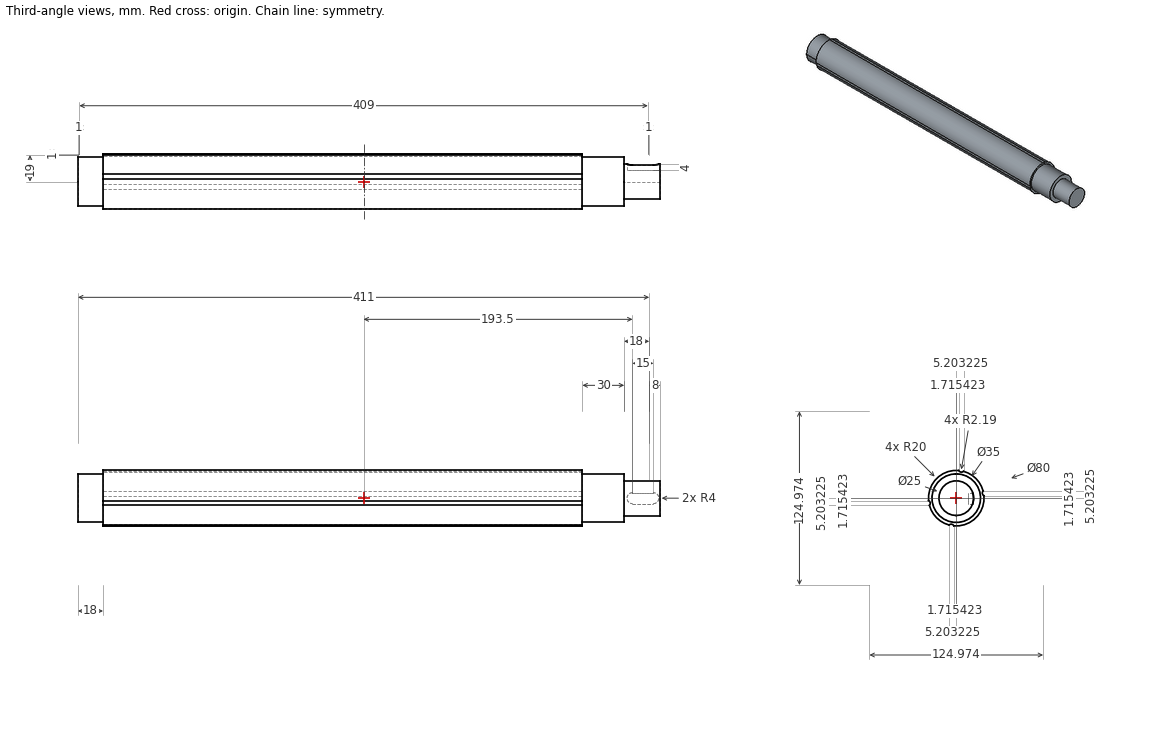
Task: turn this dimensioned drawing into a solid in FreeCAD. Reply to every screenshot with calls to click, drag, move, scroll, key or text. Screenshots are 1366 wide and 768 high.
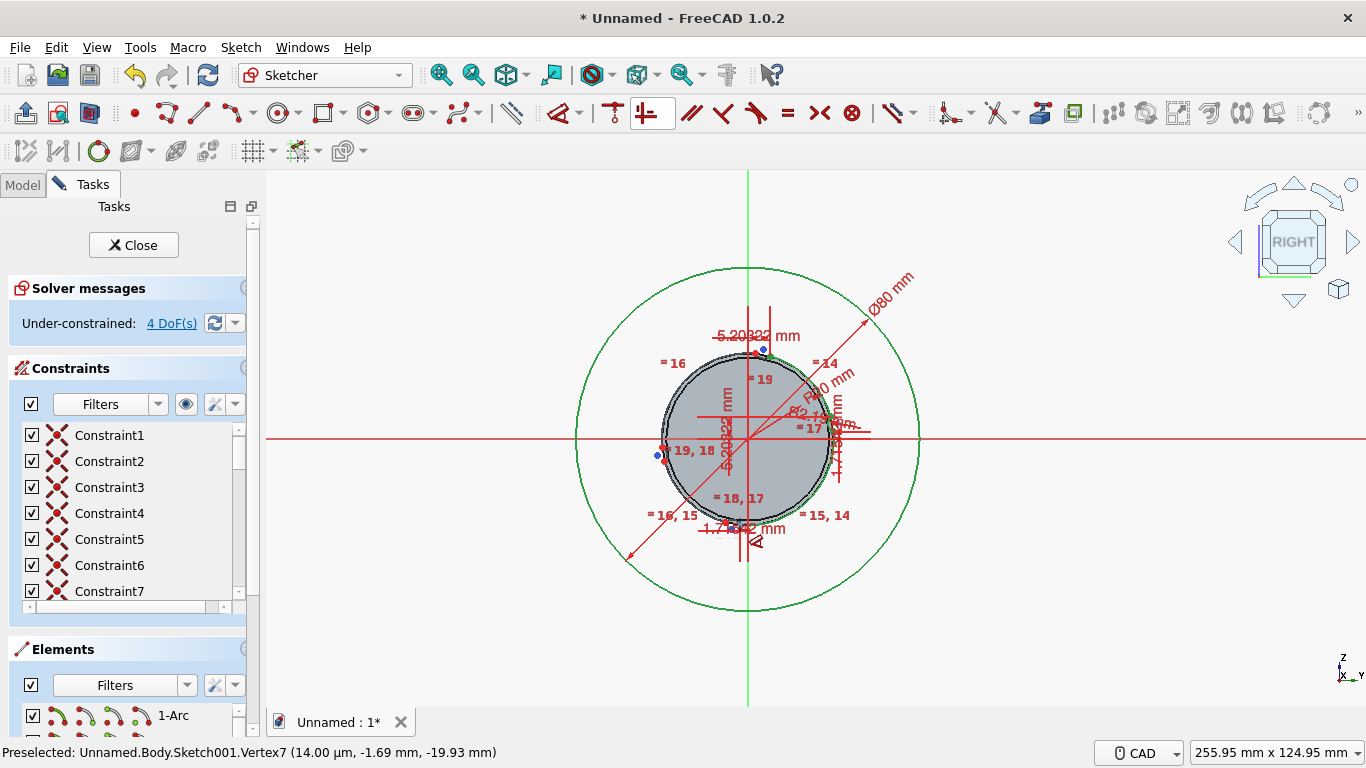
scroll(725, 522, up, 3)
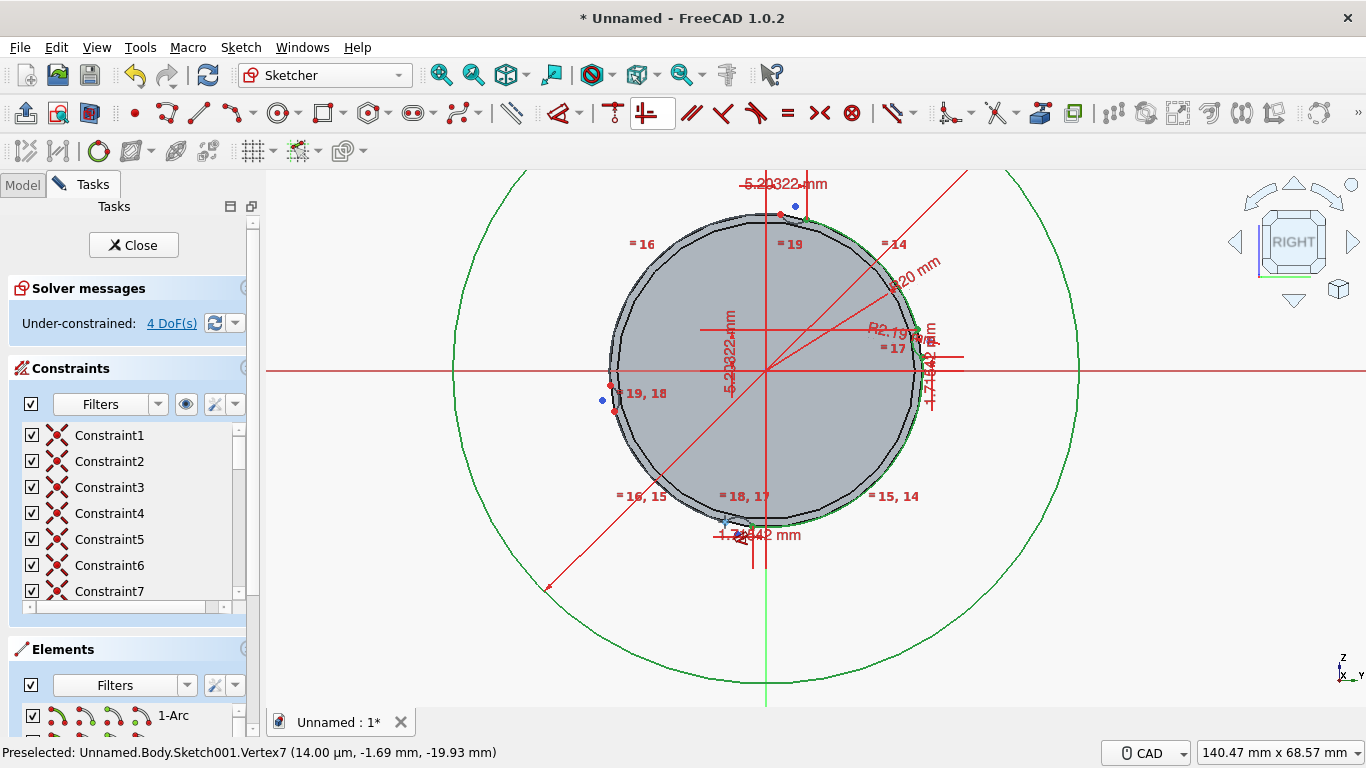
click(726, 522)
click(746, 580)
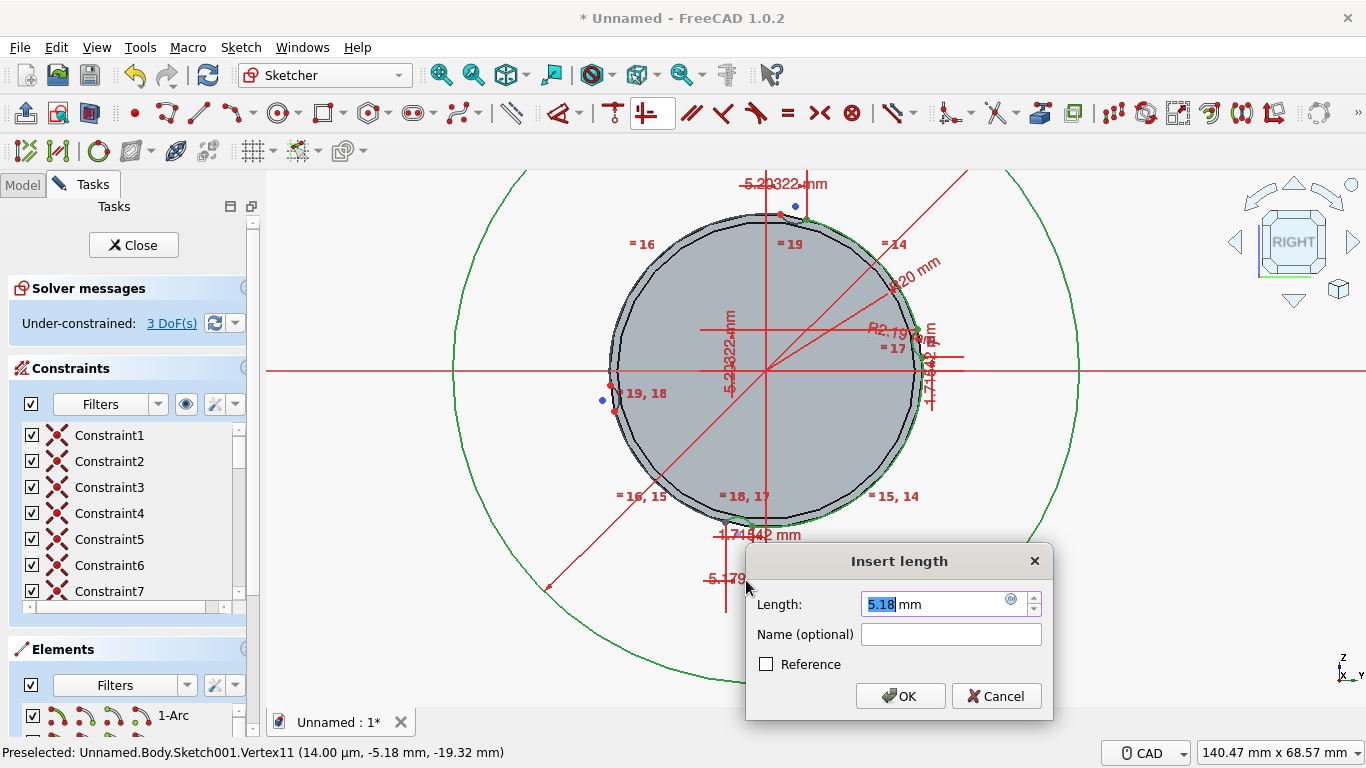
text(5.203225)
key(Return)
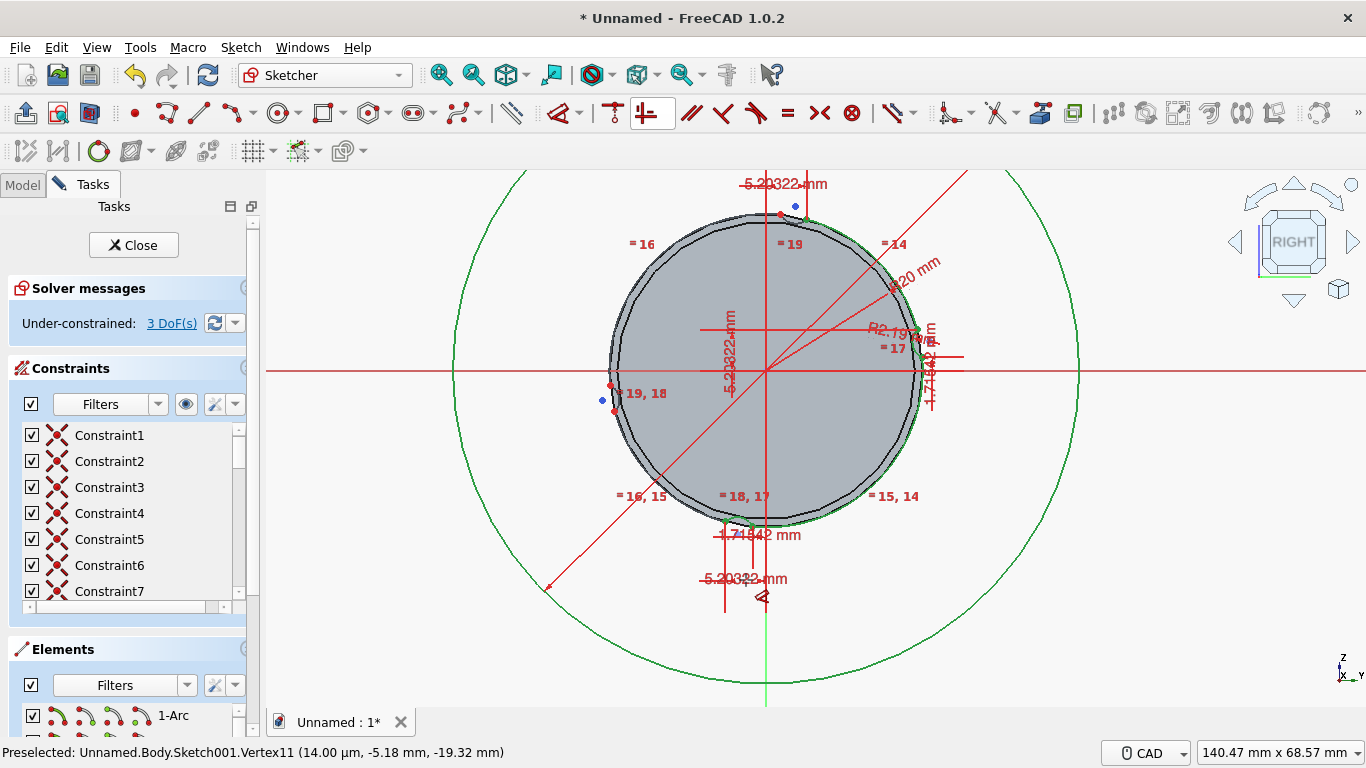
click(615, 412)
click(581, 391)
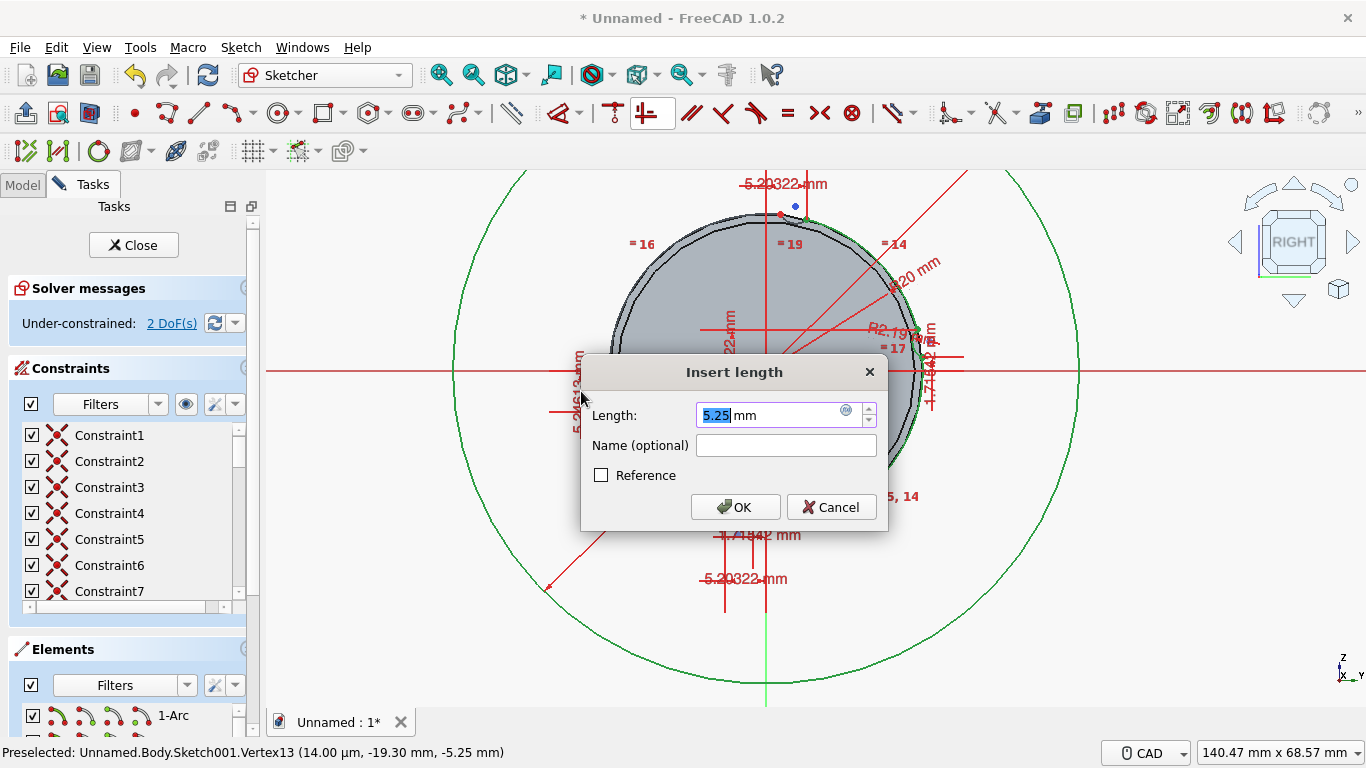
text(5.203225)
key(Return)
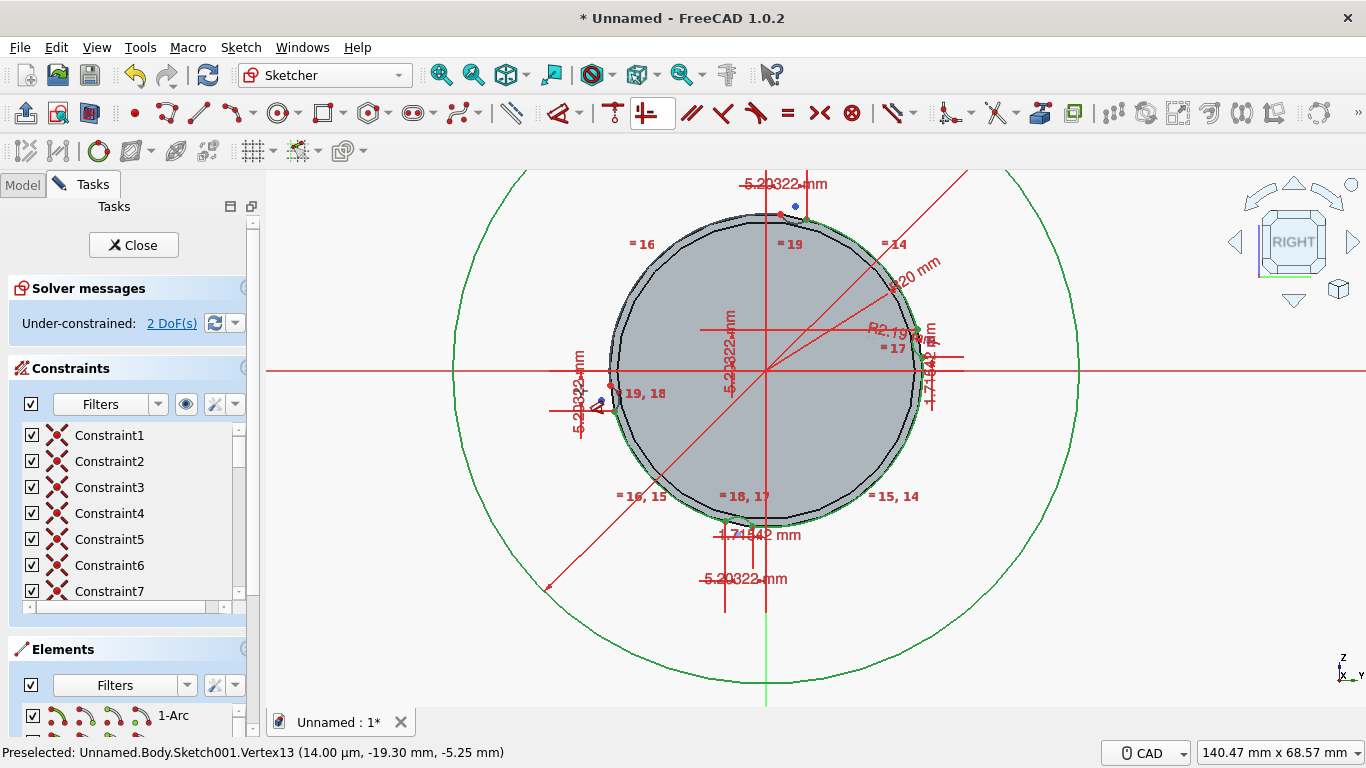
scroll(610, 385, up, 6)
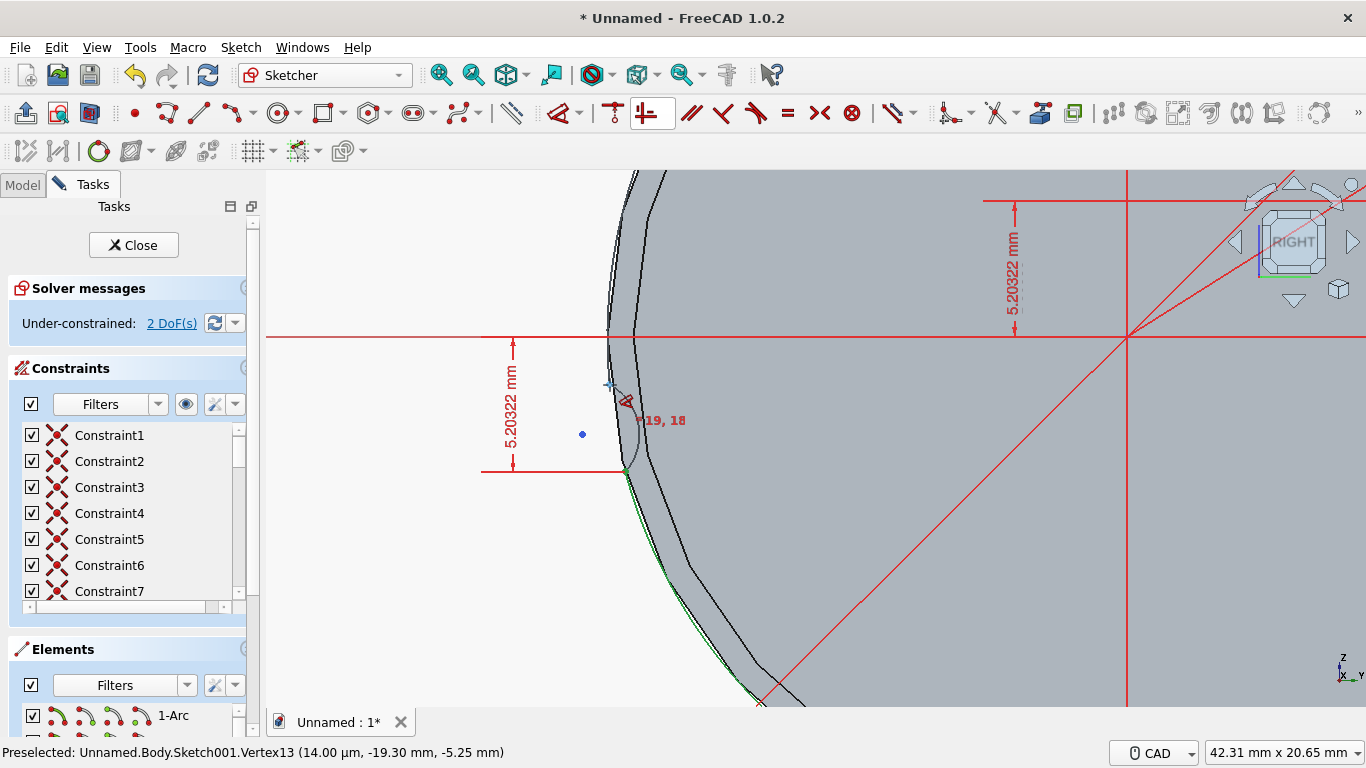
click(610, 385)
click(576, 361)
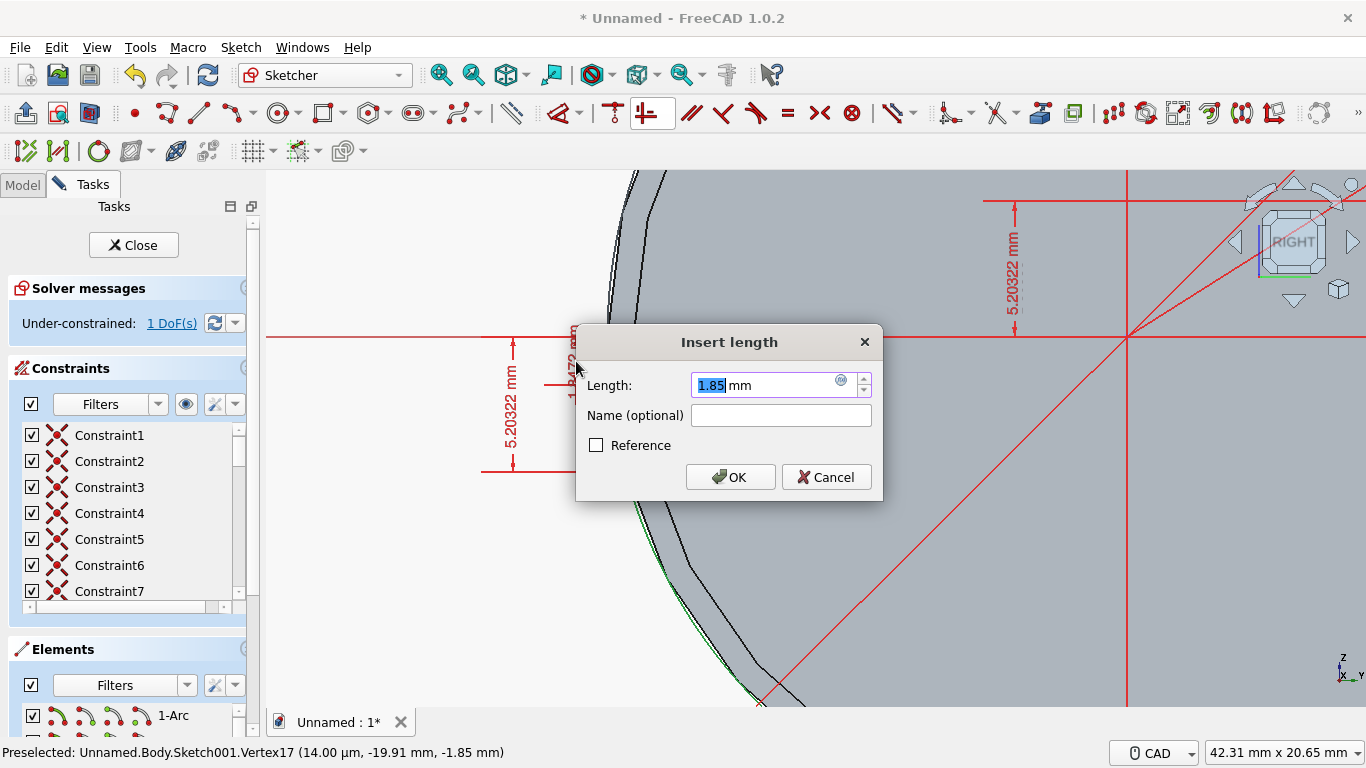
text(1.715423)
key(Return)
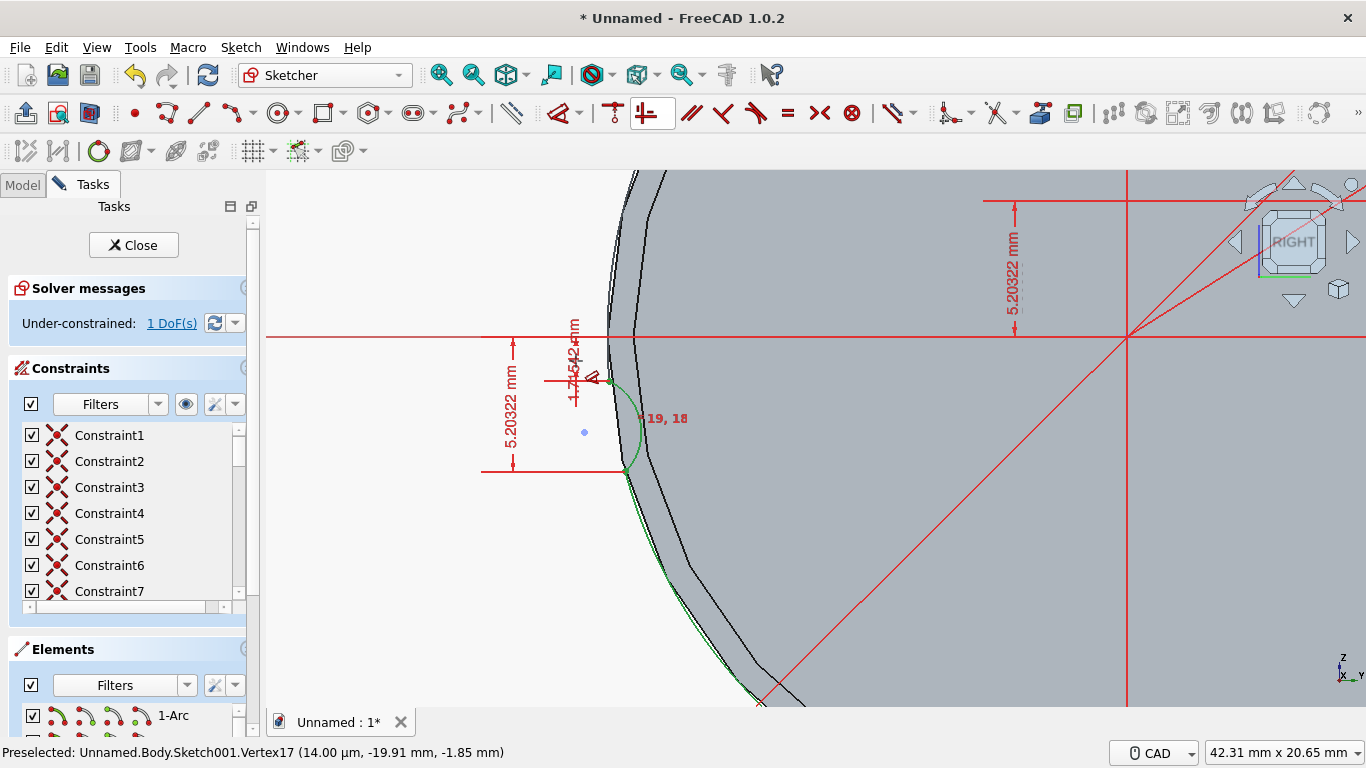
scroll(672, 459, down, 9)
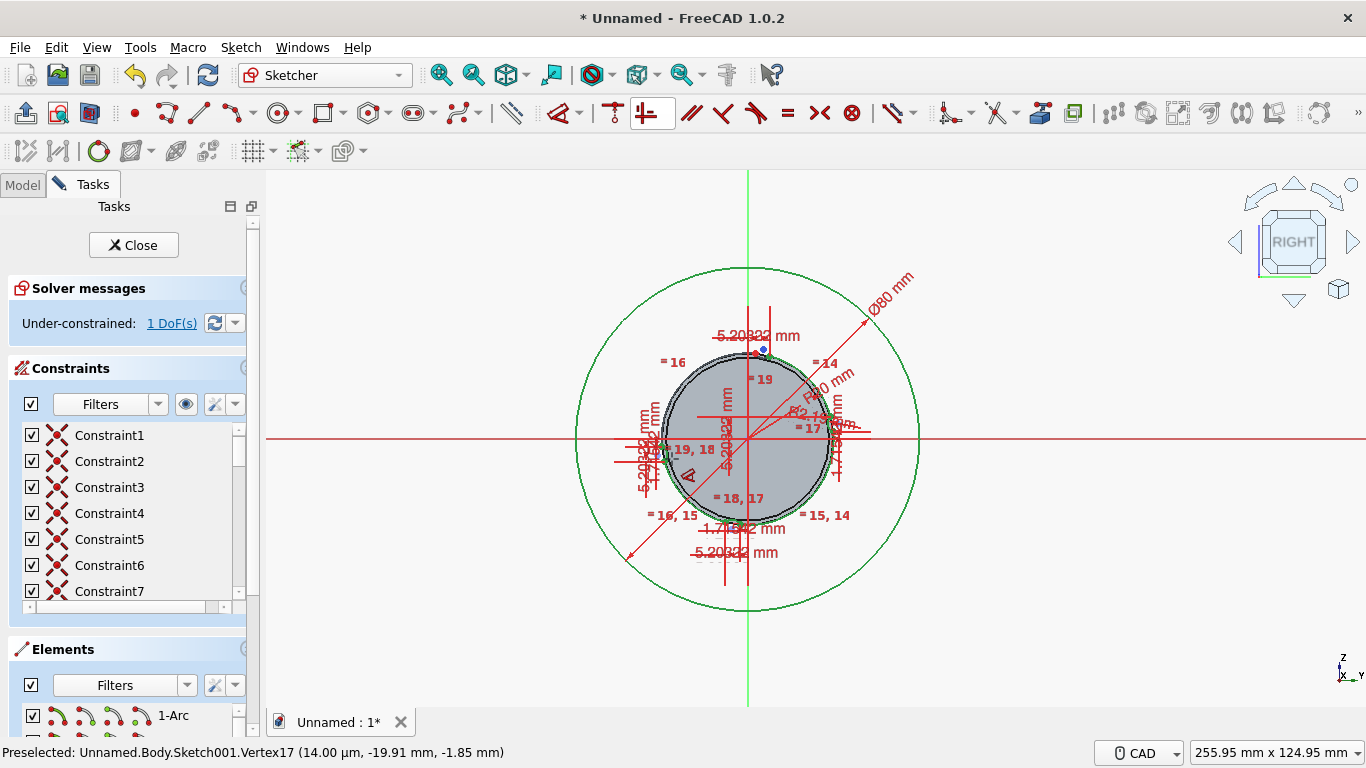
scroll(756, 354, up, 9)